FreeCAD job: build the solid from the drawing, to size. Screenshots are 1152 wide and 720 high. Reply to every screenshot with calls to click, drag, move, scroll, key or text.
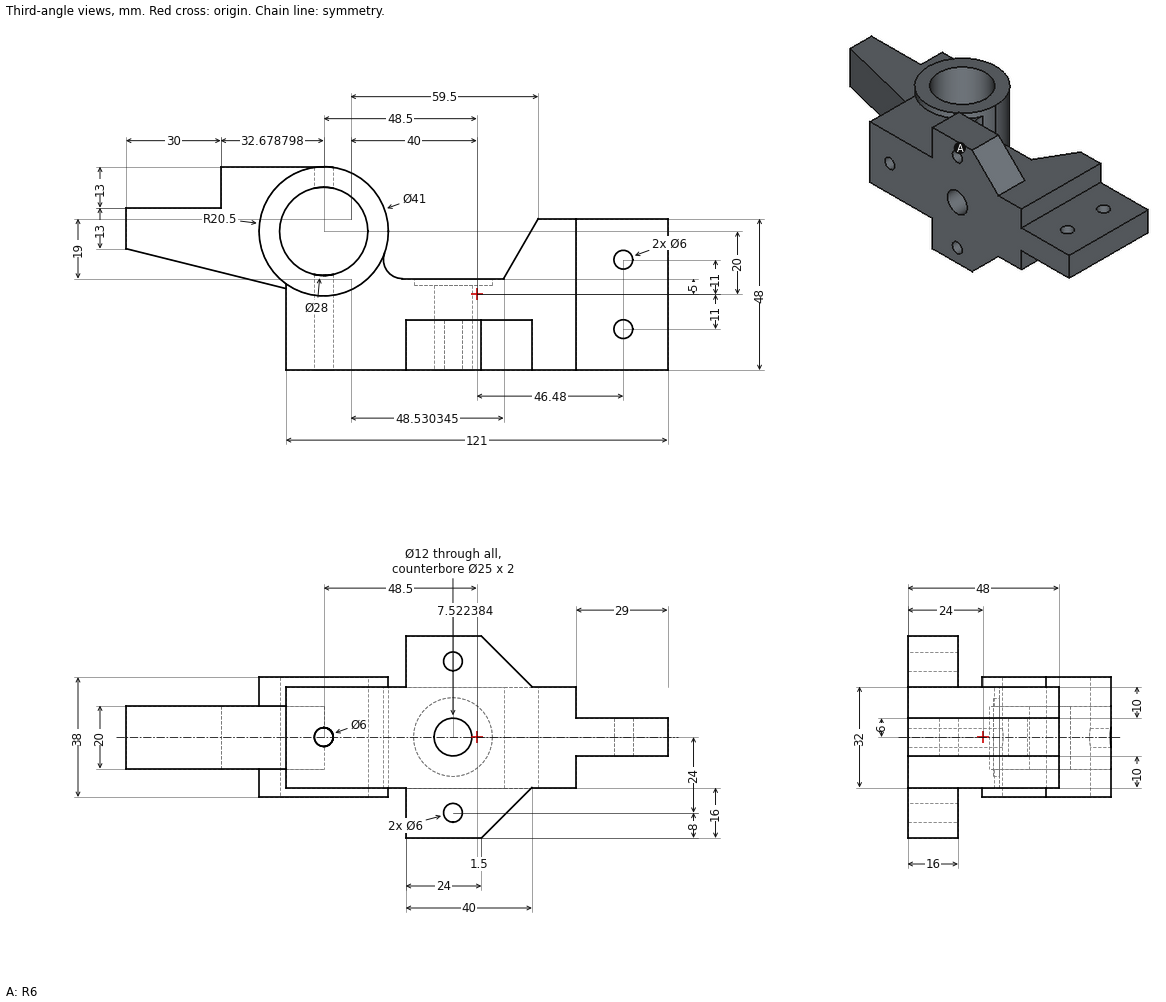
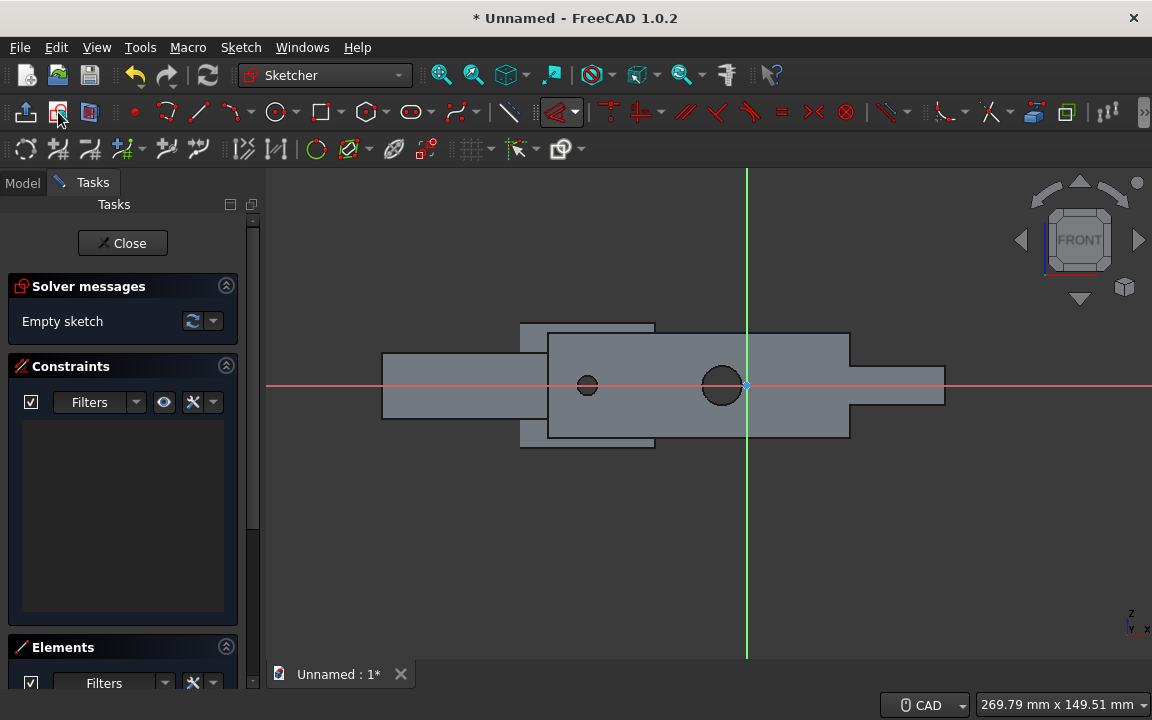
scroll(938, 329, up, 2)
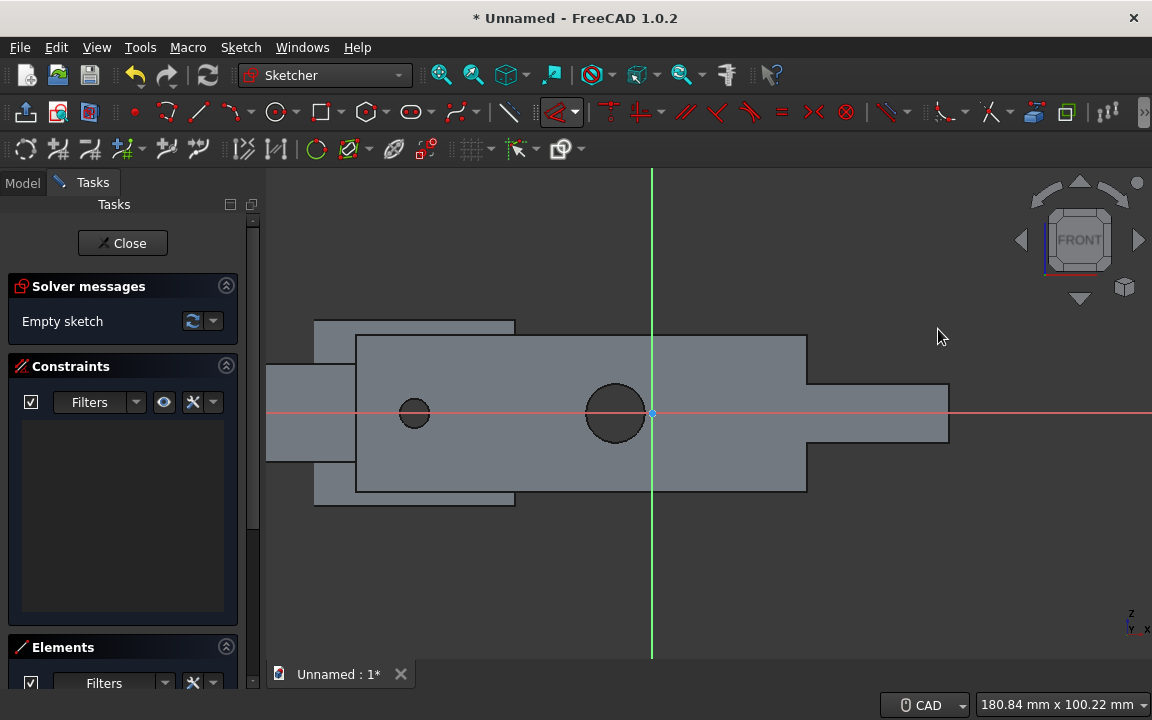
click(168, 112)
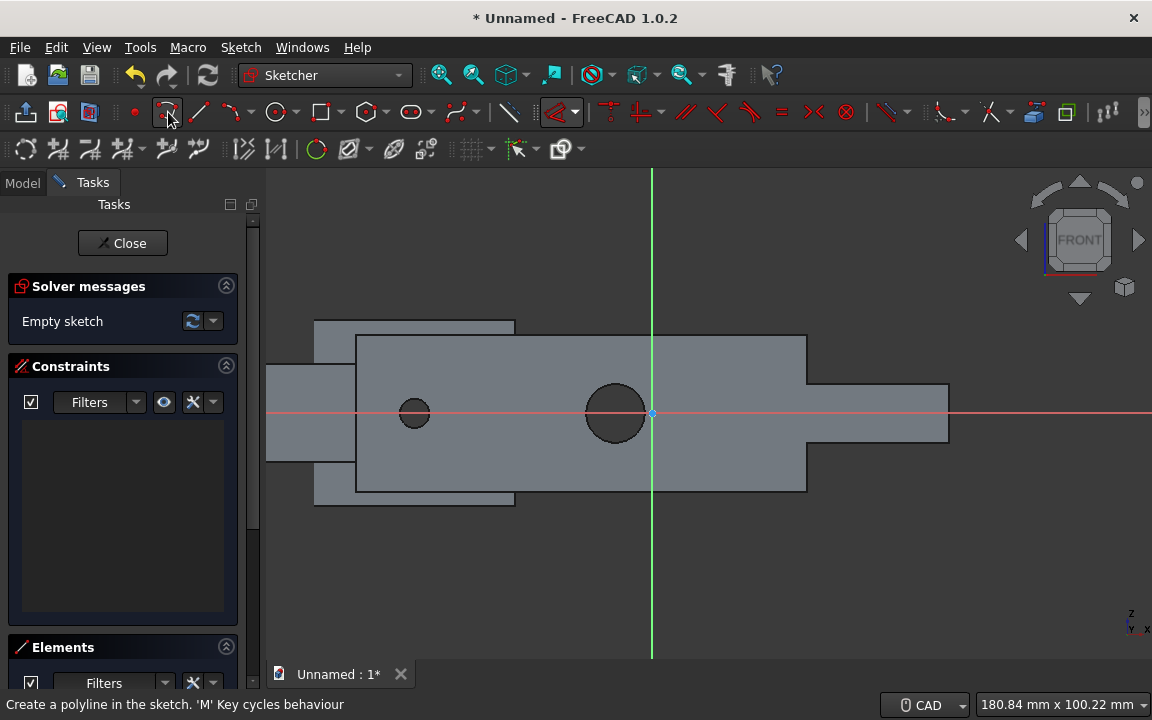
click(738, 492)
click(542, 492)
click(542, 570)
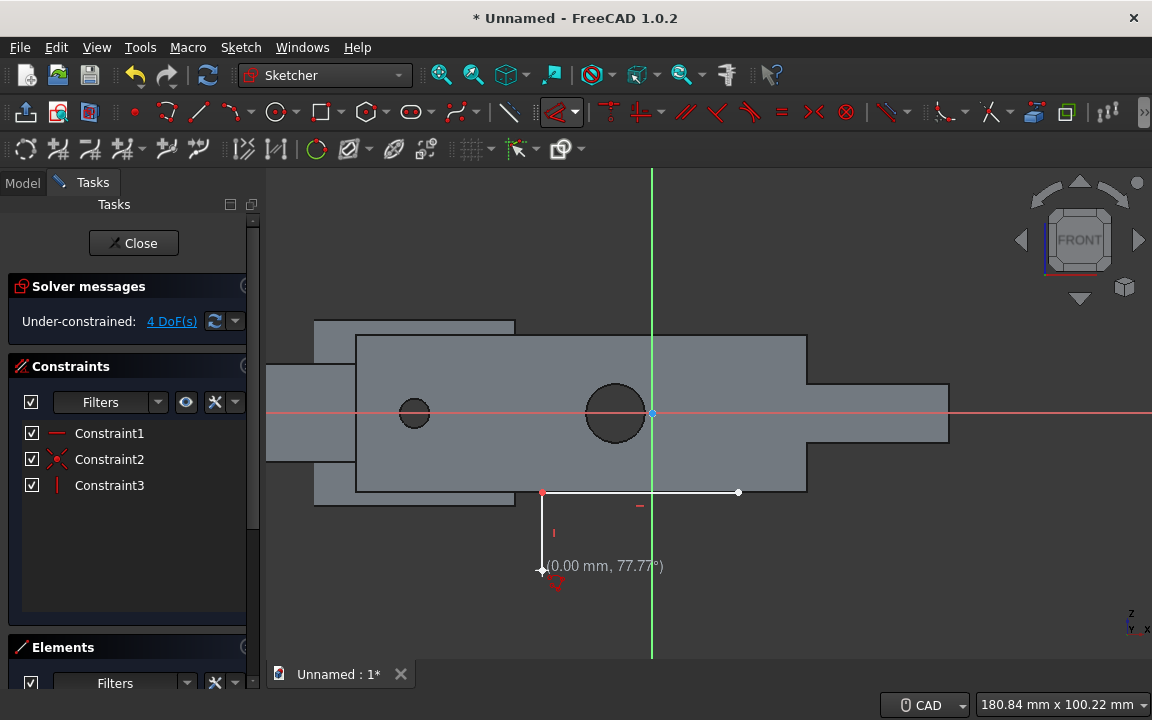
scroll(660, 570, up, 4)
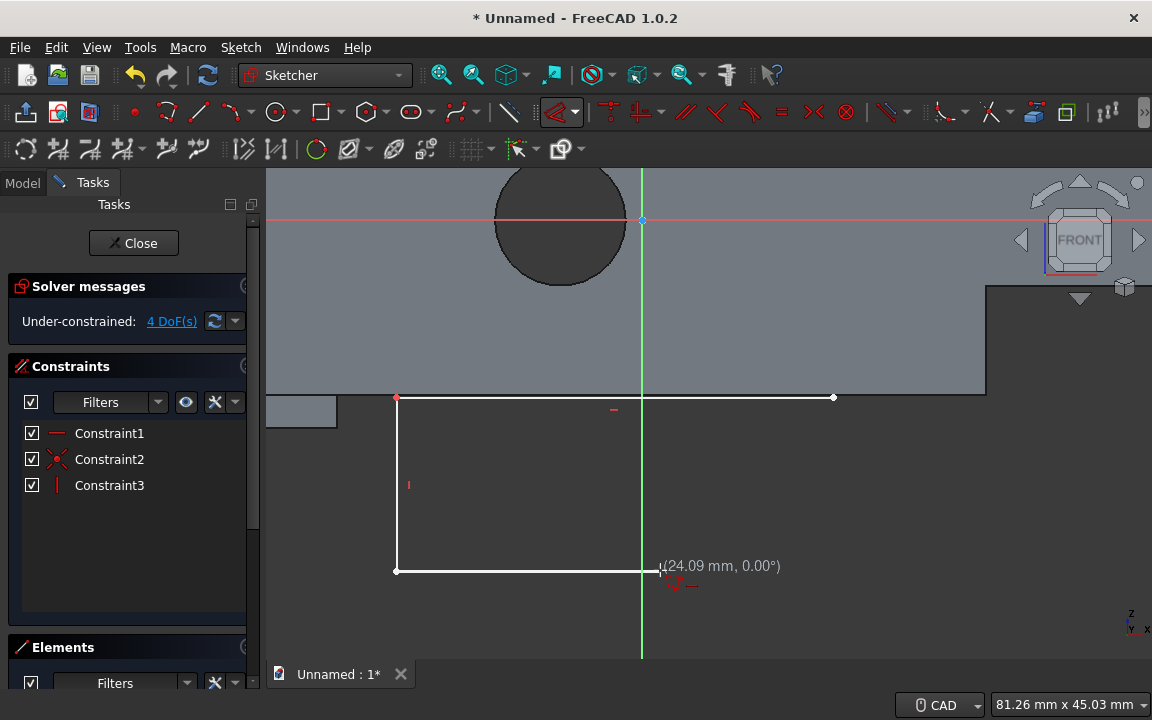
click(659, 569)
click(833, 398)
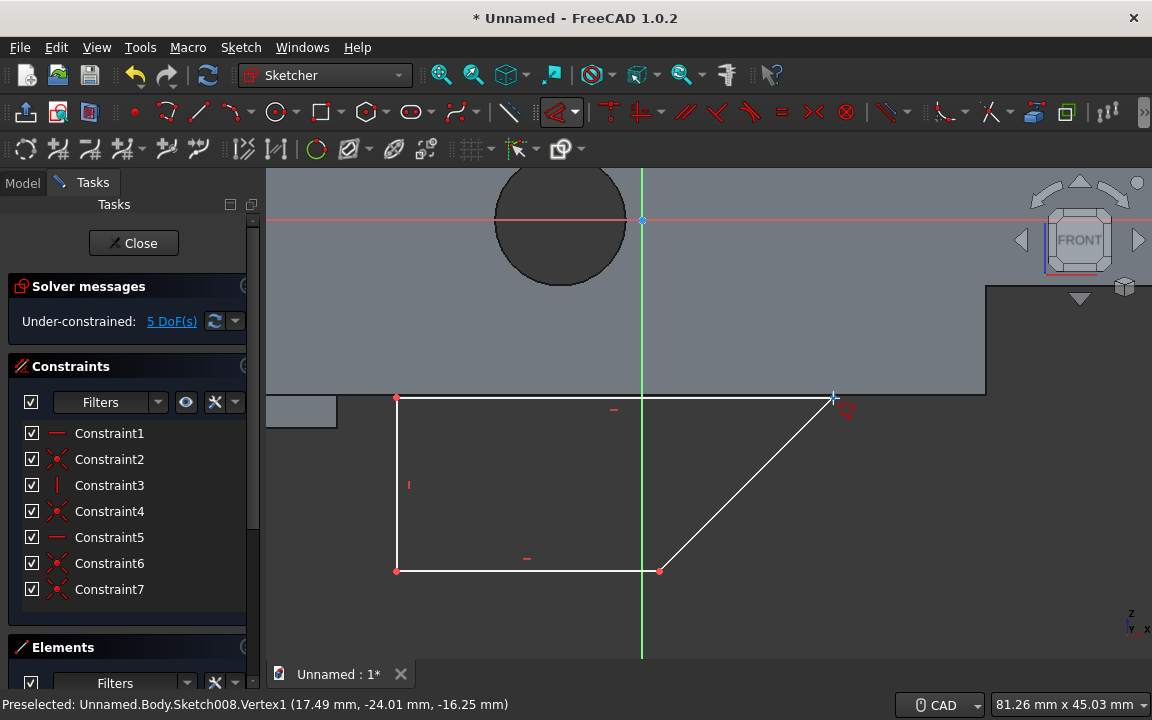
scroll(661, 571, down, 4)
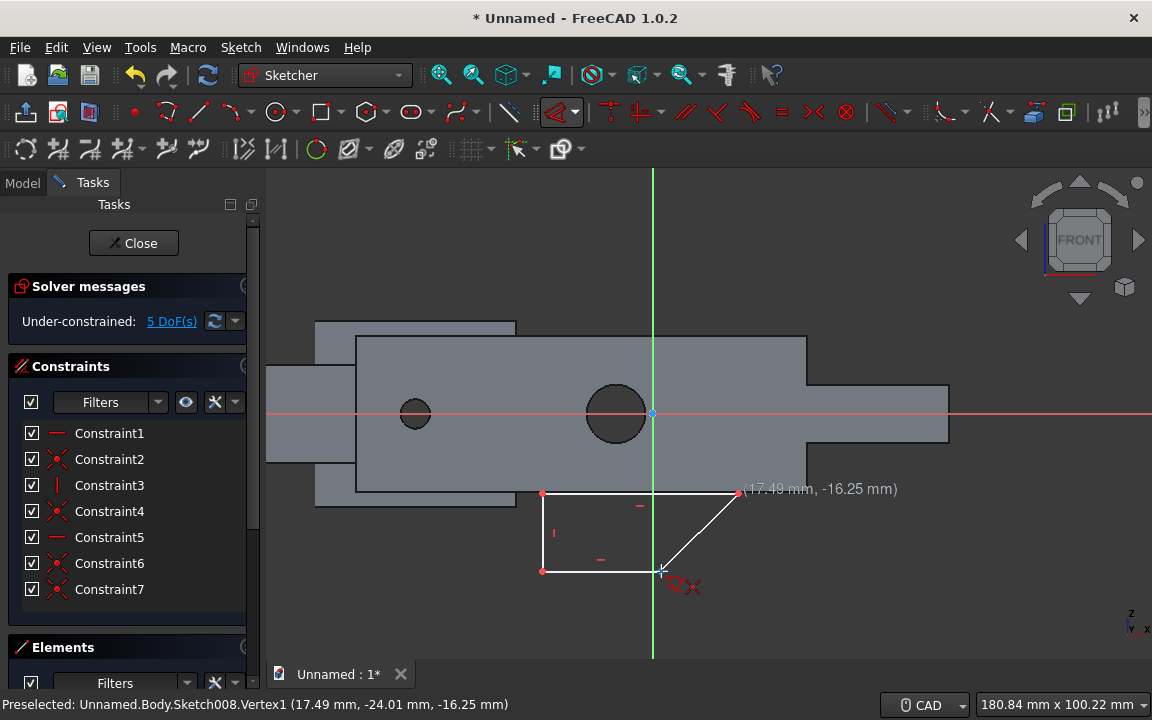
click(739, 336)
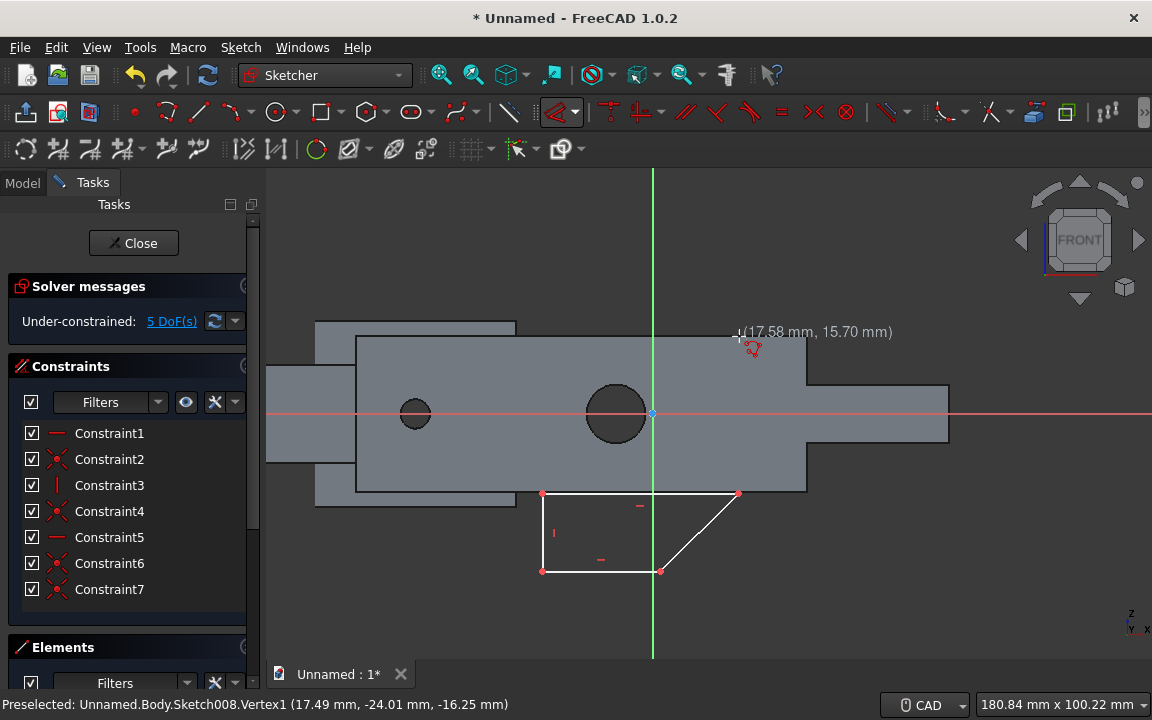
scroll(660, 257, up, 4)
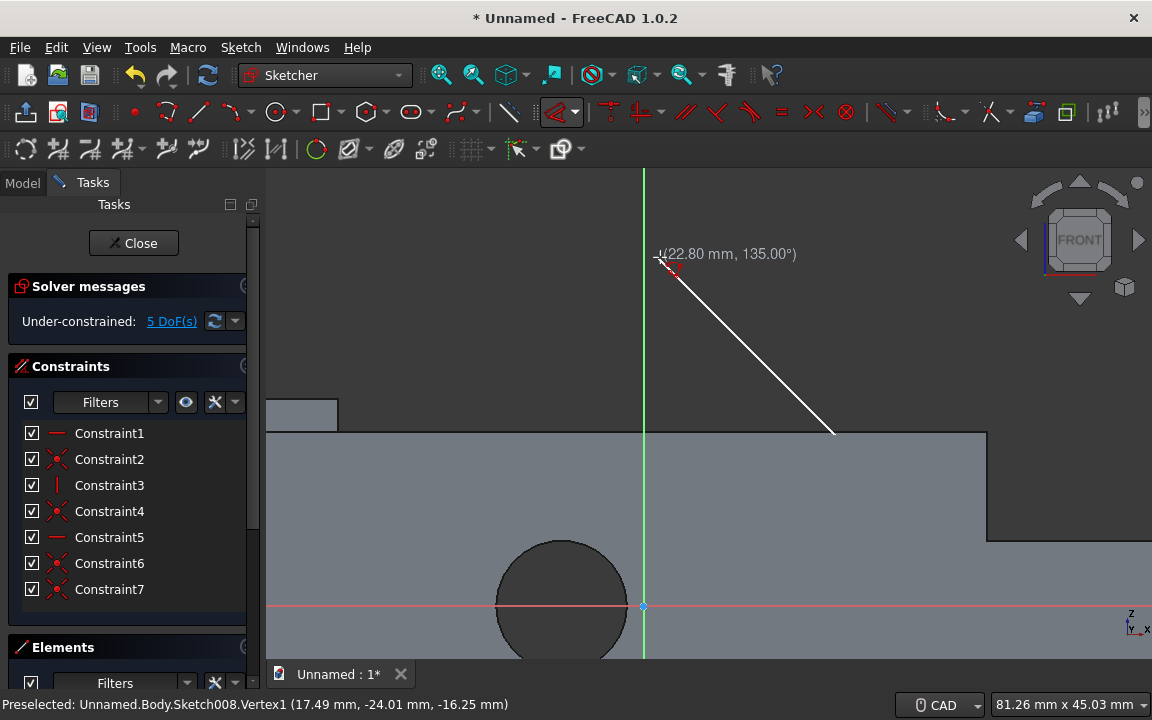
click(660, 257)
click(398, 257)
click(398, 432)
click(835, 435)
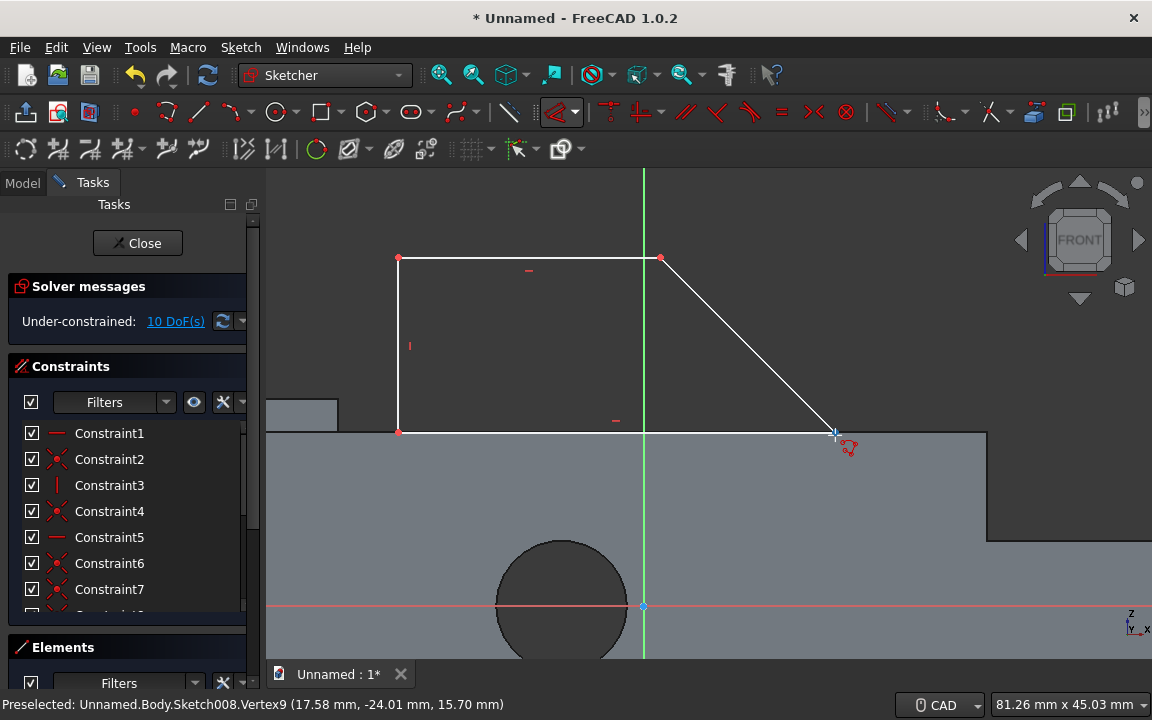
key(g)
key(c)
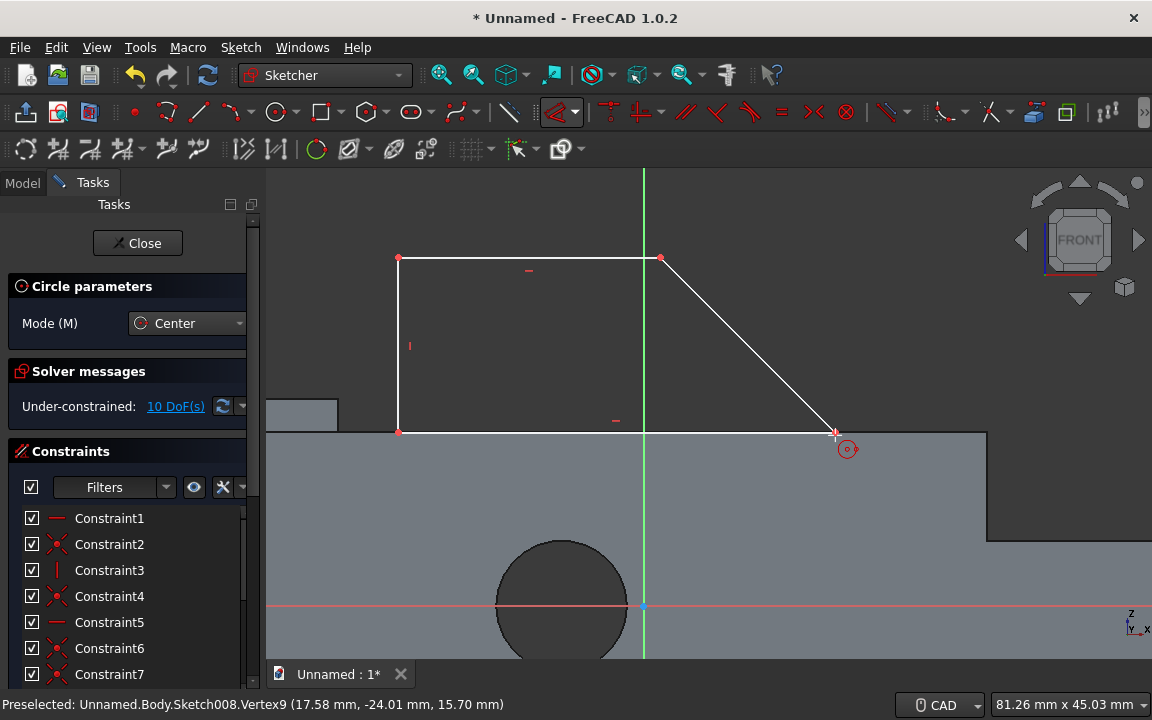
scroll(660, 256, down, 4)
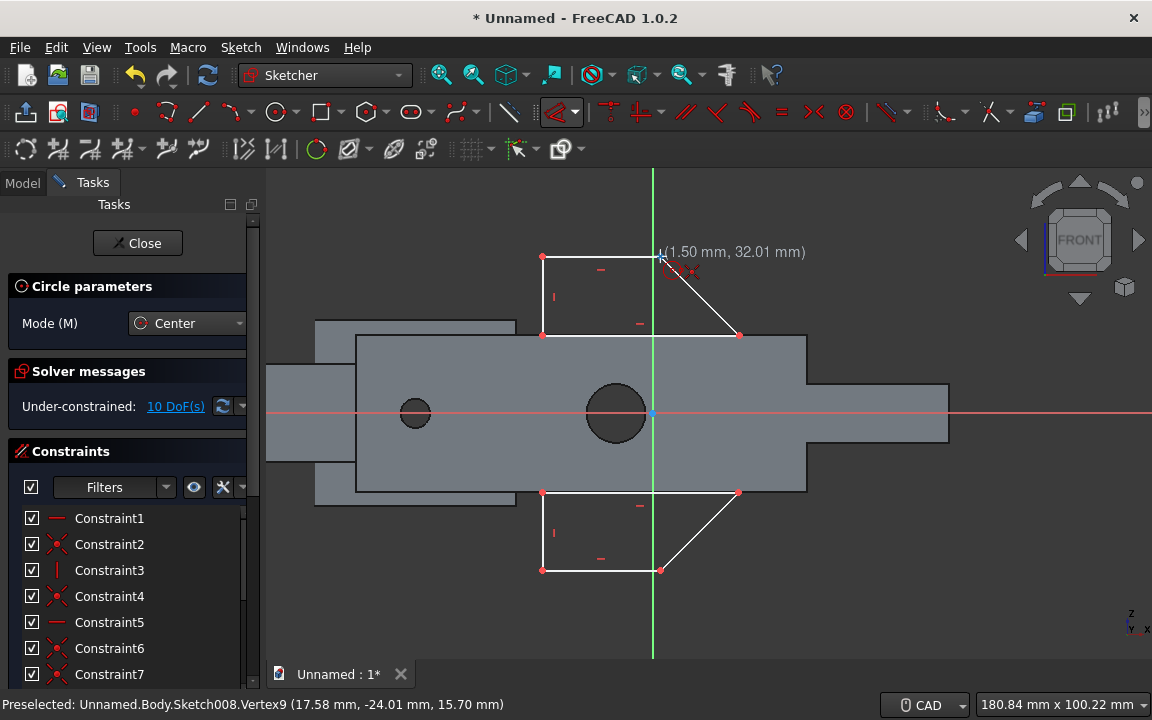
scroll(616, 531, up, 3)